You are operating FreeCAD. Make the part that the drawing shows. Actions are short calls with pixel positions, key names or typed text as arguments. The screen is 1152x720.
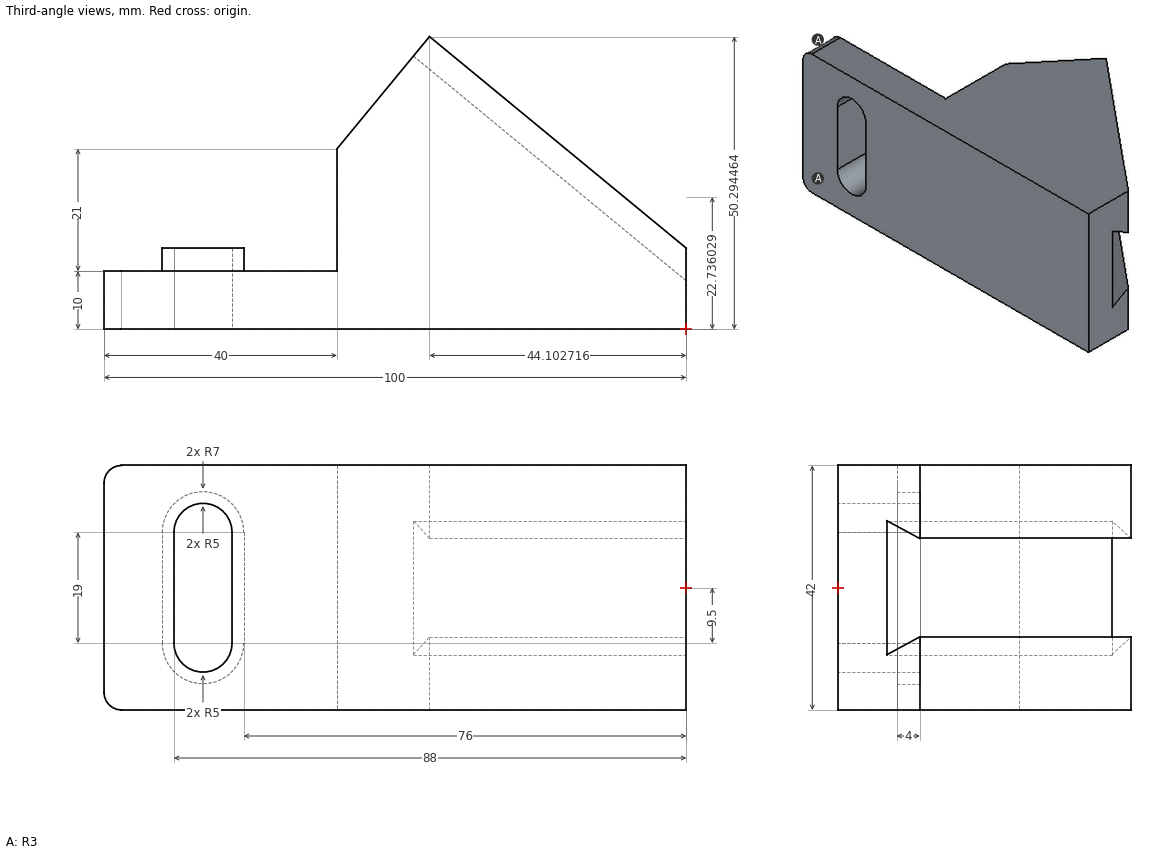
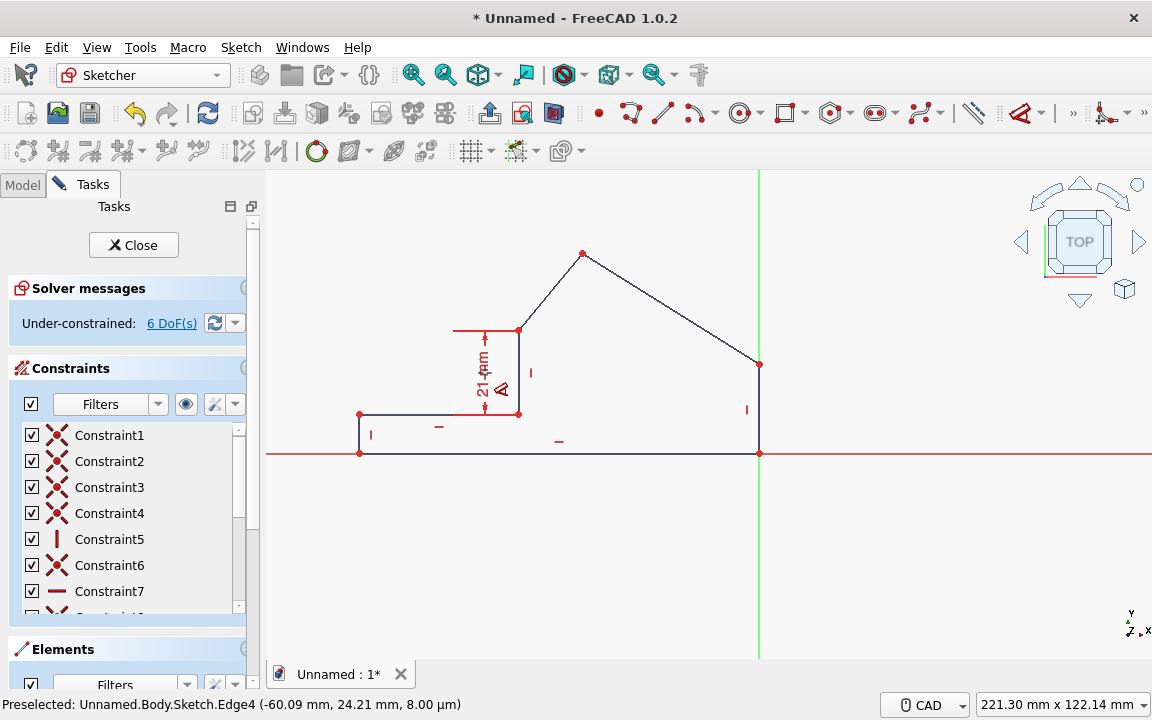
click(471, 415)
click(402, 381)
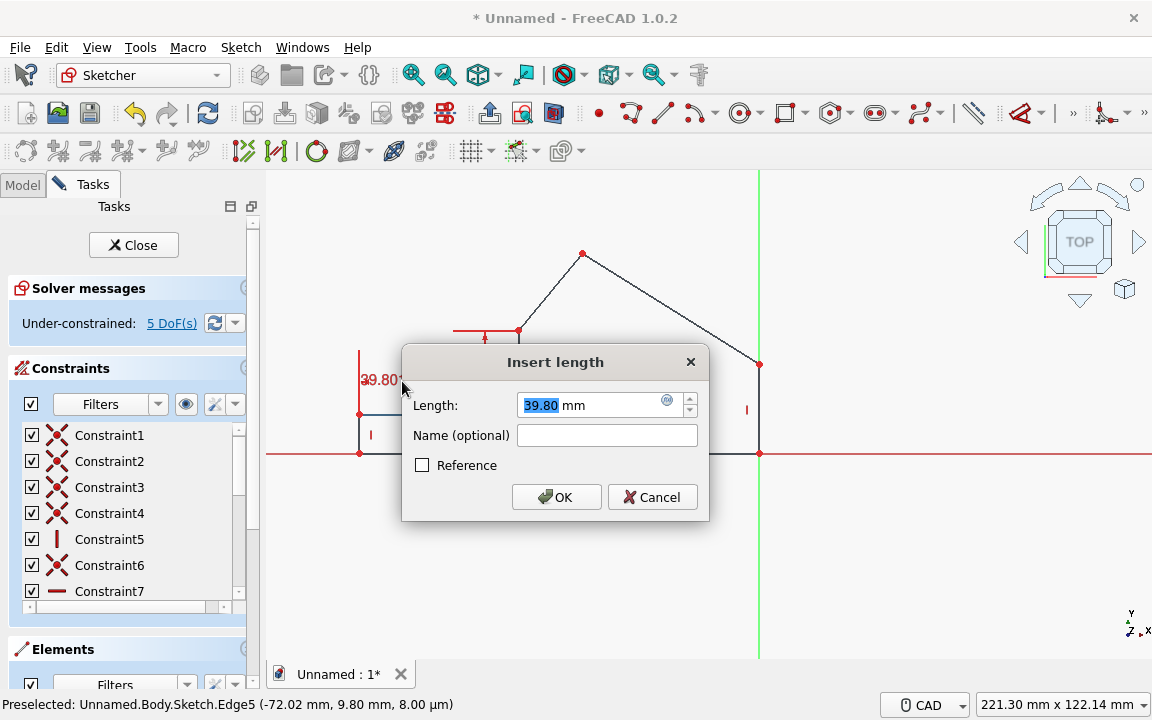
text(40)
key(Return)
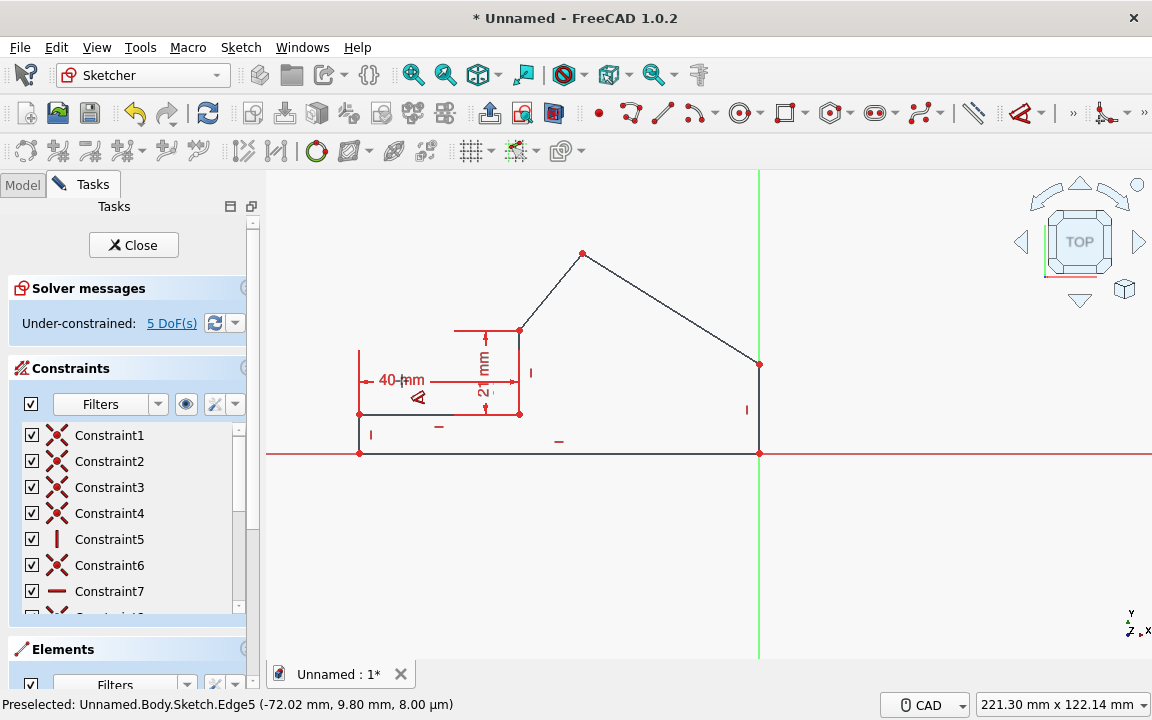
click(359, 426)
click(325, 434)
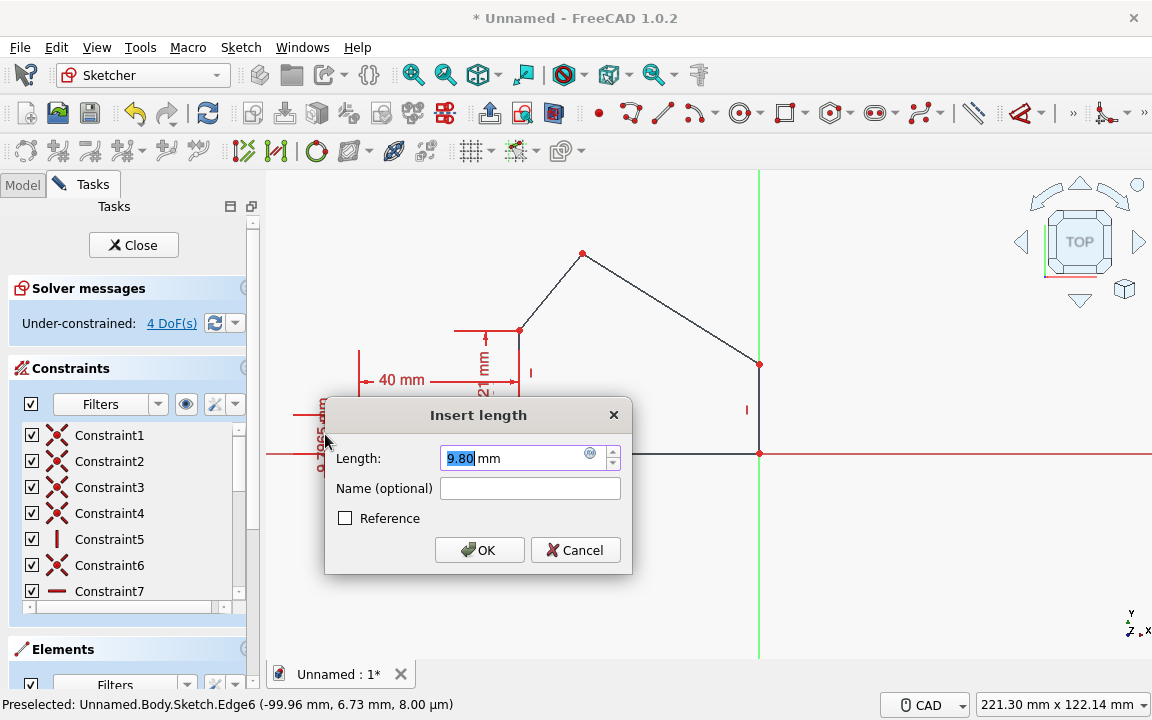
text(10)
key(Return)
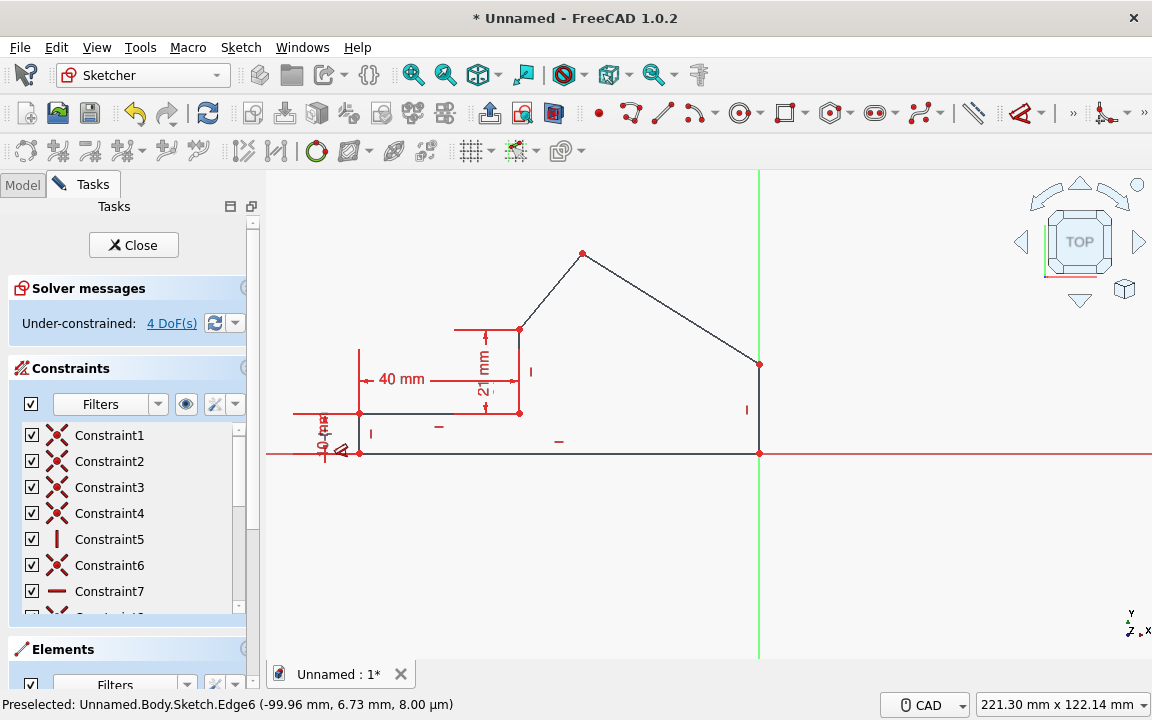
click(479, 454)
click(559, 488)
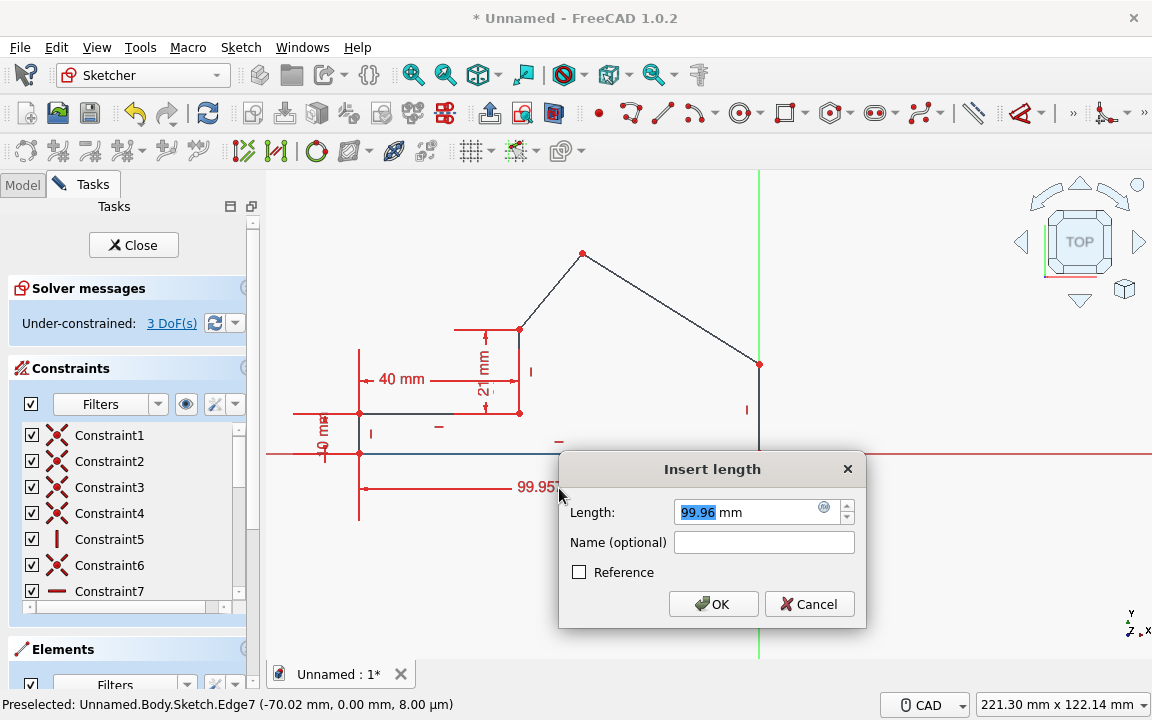
text(100)
key(Return)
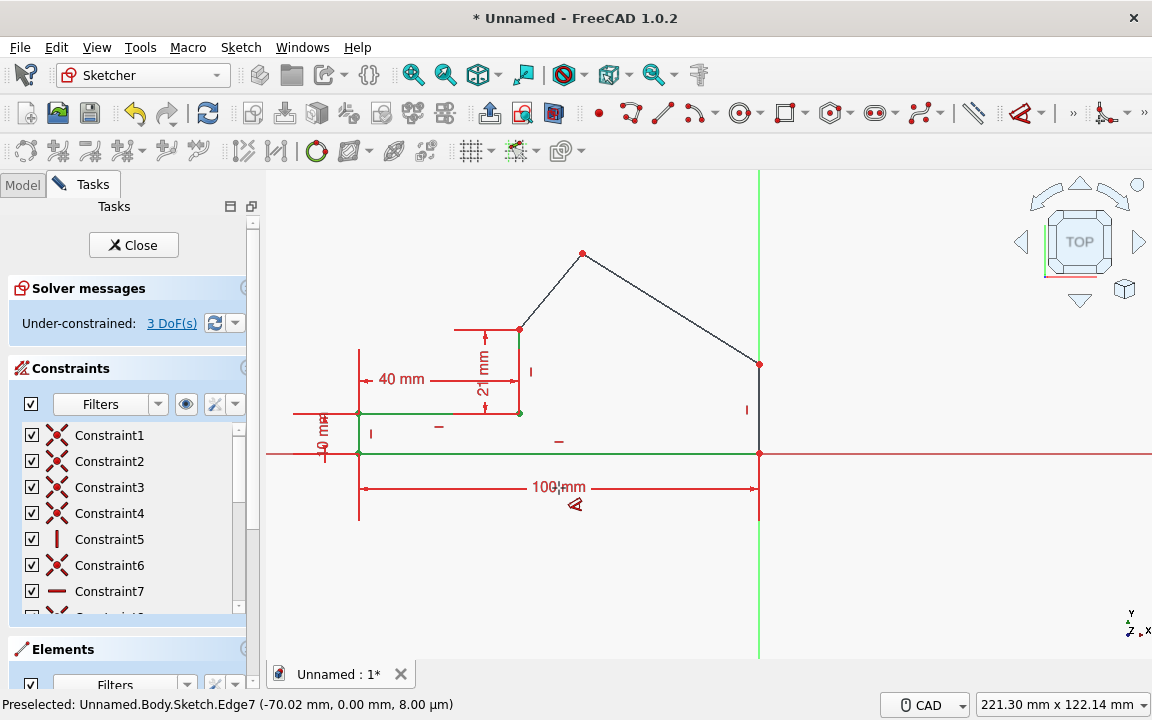
click(759, 427)
click(793, 409)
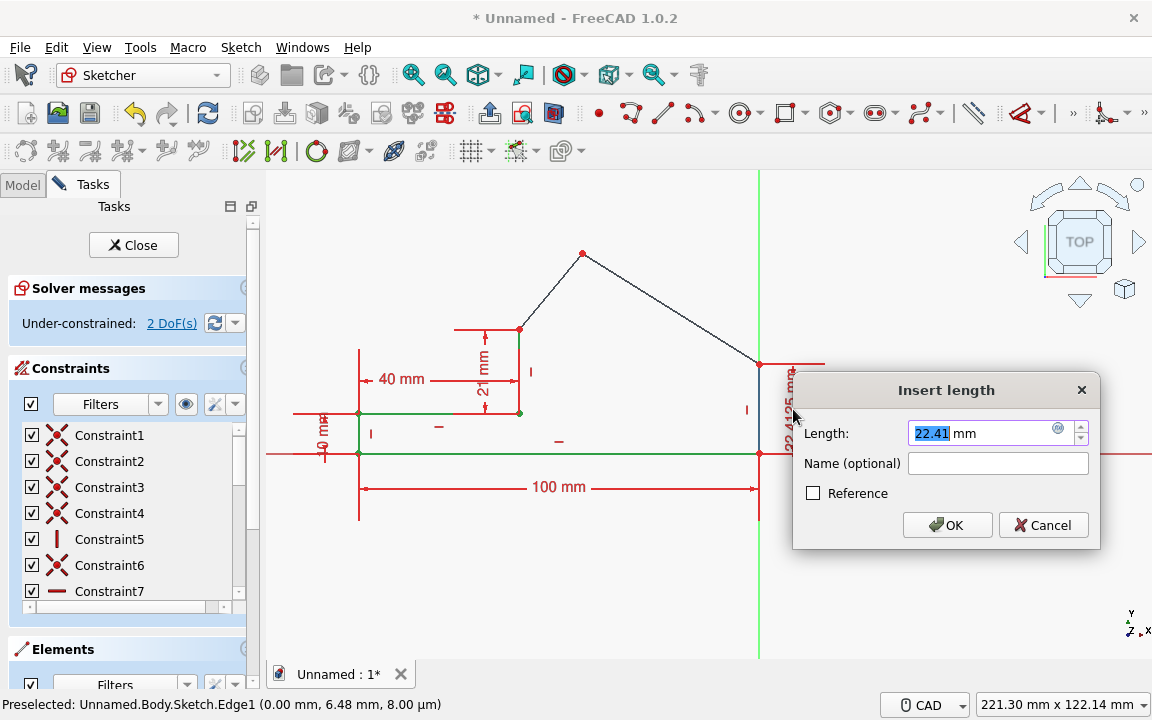
text(22.736029)
key(Return)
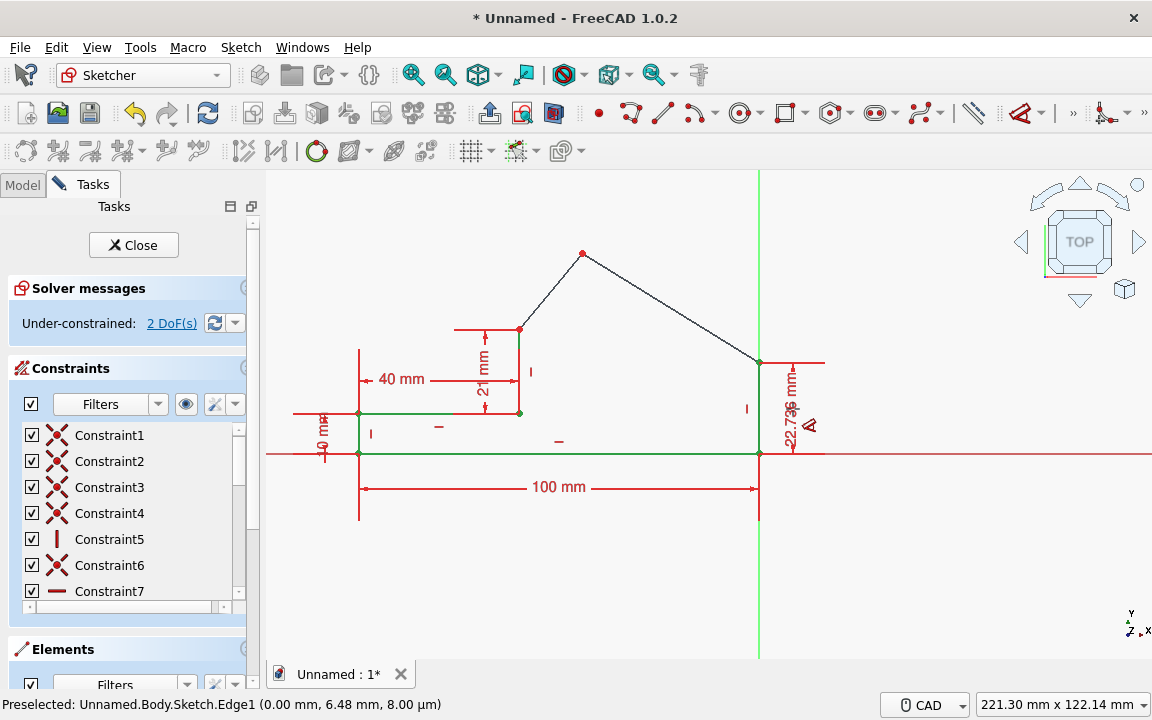
click(583, 254)
click(671, 488)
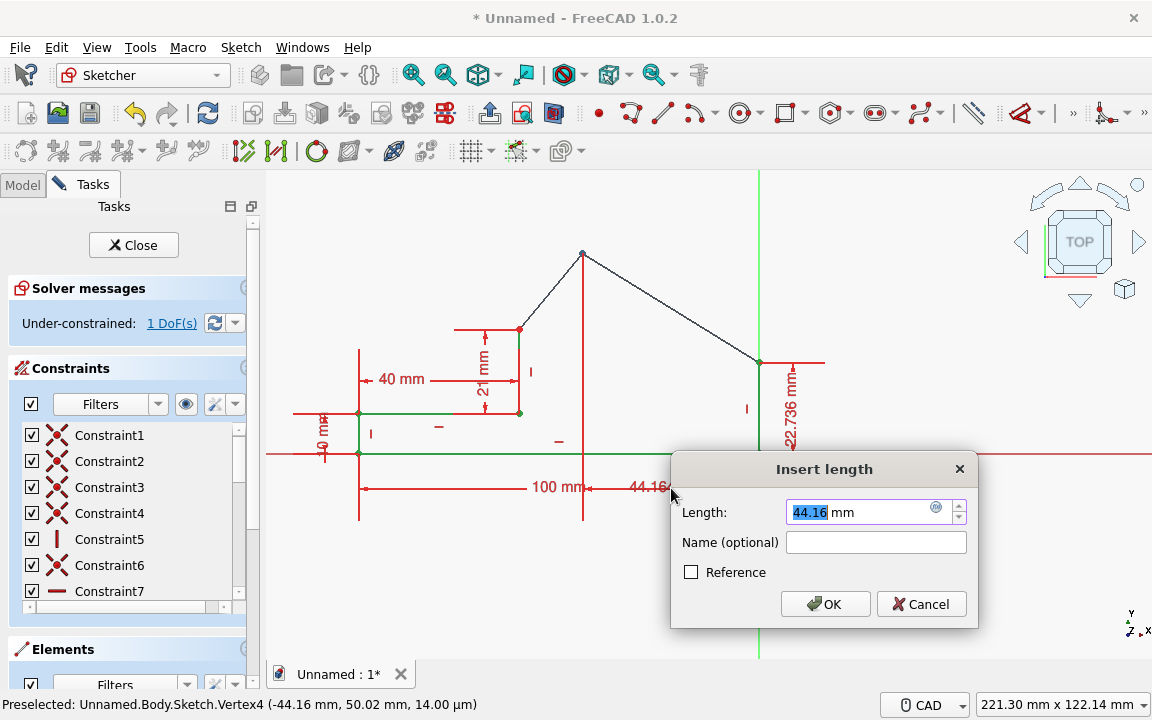
text(44.102716)
key(Return)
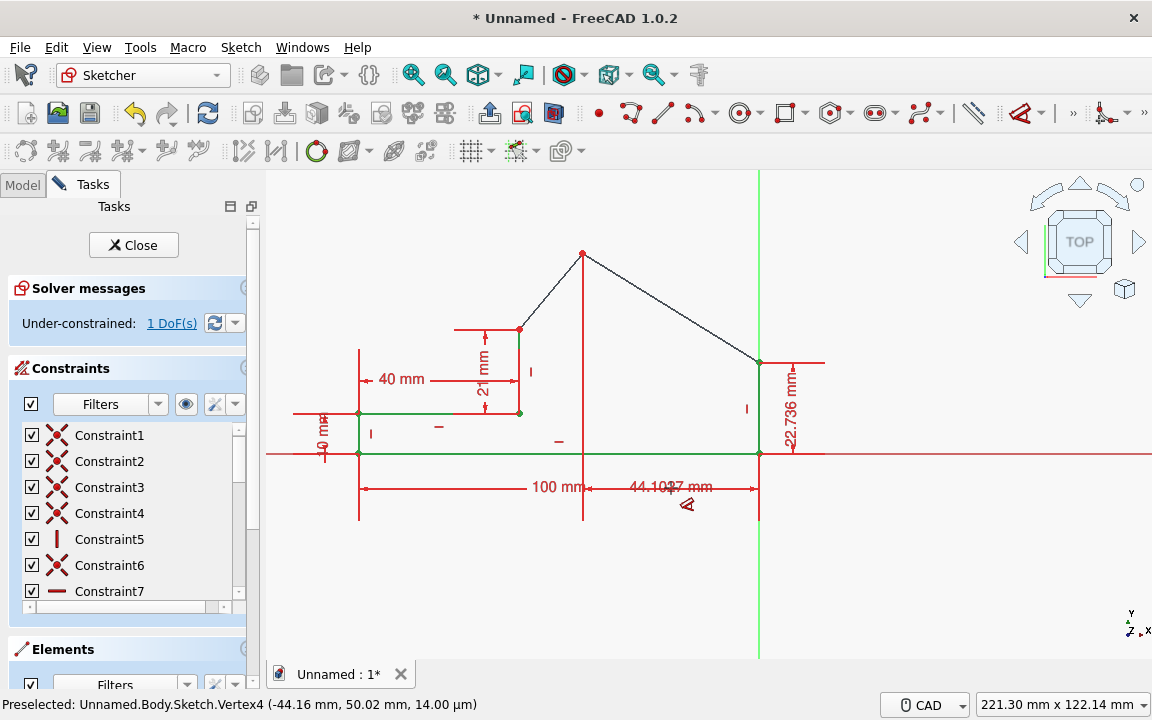
click(583, 254)
click(793, 354)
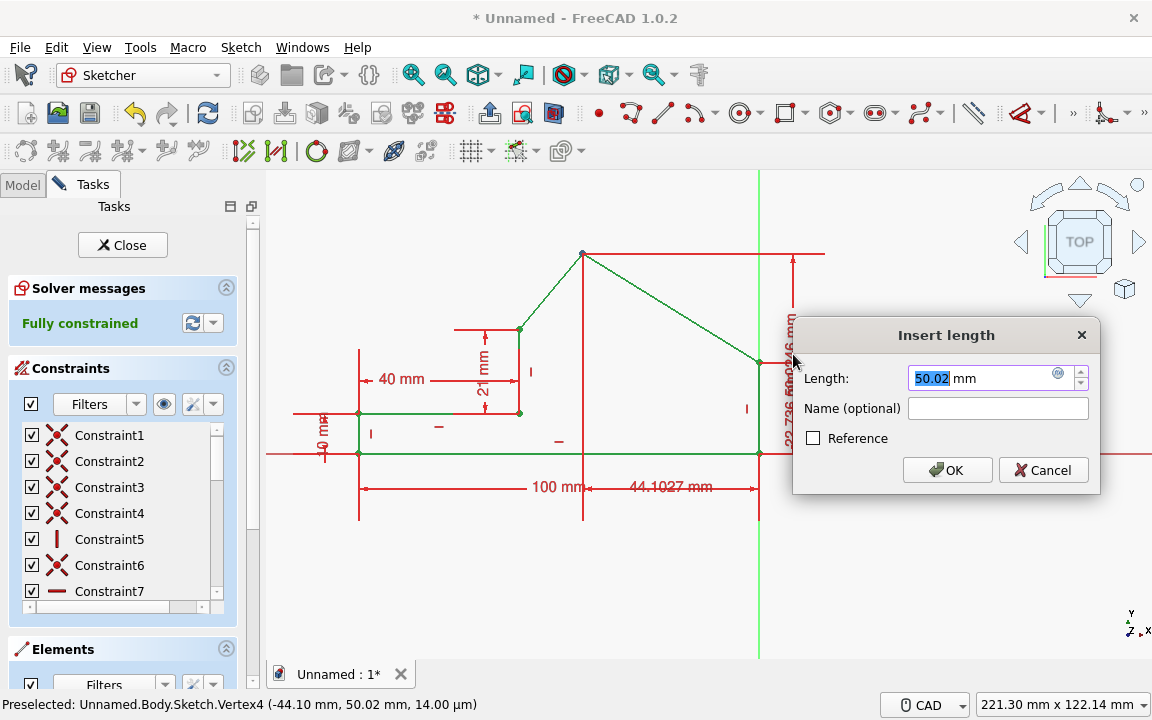
text(50.294464)
key(Return)
key(Escape)